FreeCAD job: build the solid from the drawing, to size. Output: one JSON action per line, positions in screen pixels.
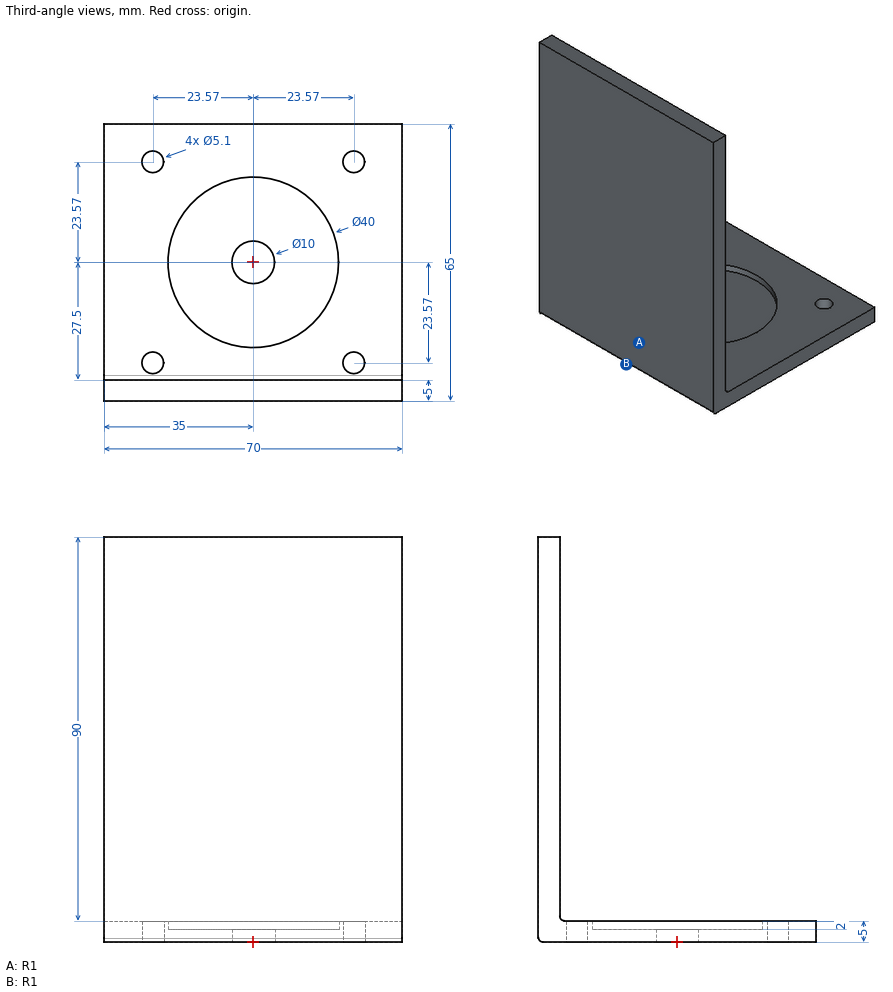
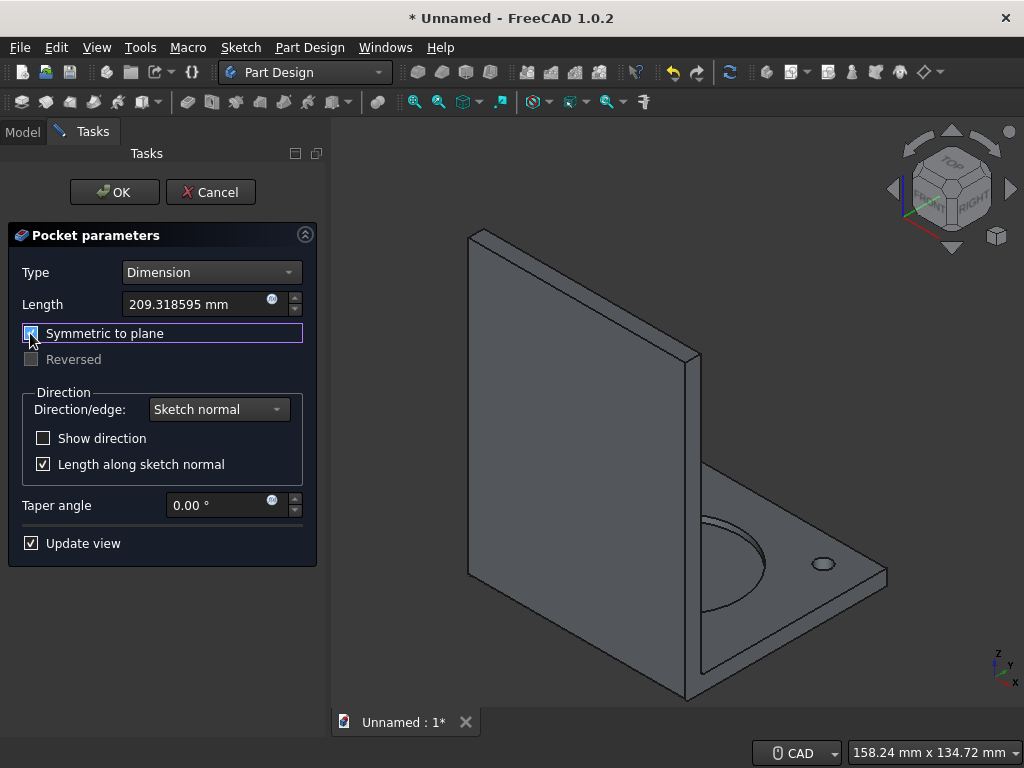
{"action": "left_click", "coordinate": [115, 192]}